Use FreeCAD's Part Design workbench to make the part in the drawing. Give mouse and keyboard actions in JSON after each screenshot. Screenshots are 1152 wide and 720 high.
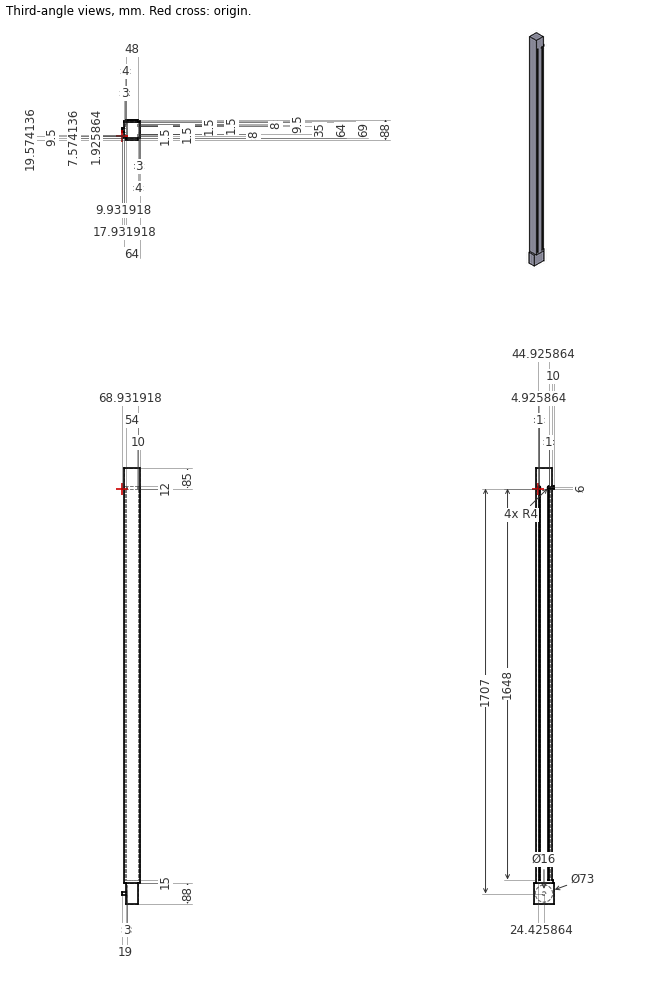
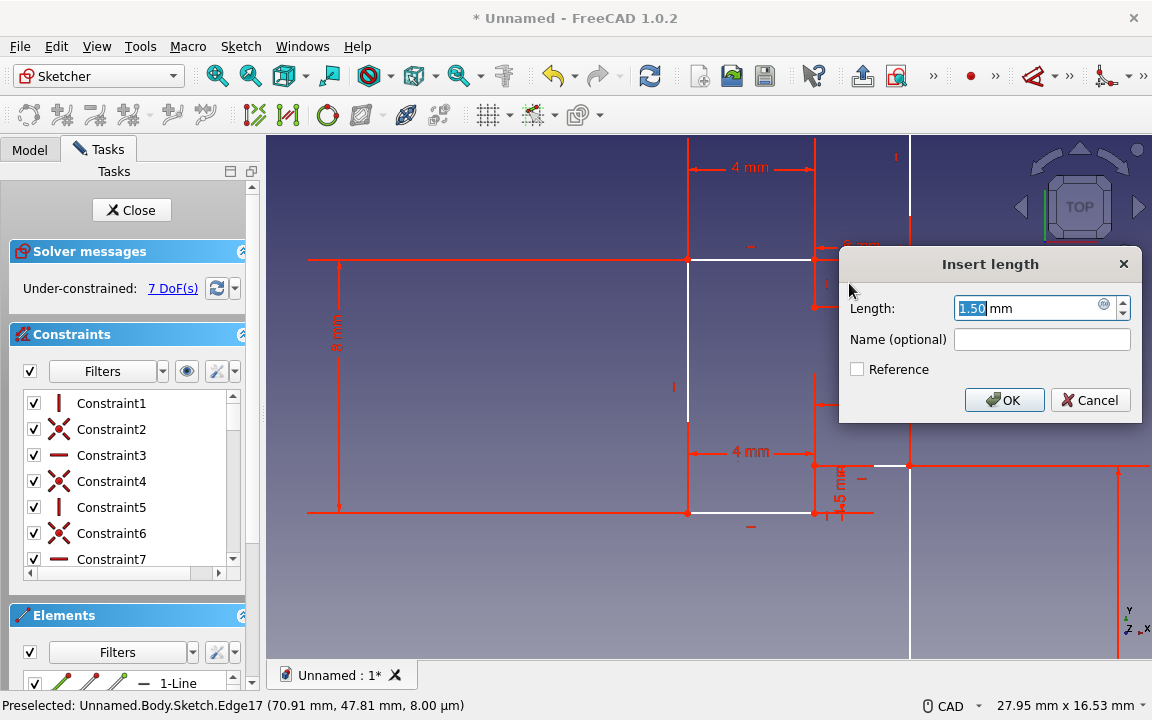
{"action": "type", "text": "1.5"}
{"action": "key", "text": "Return"}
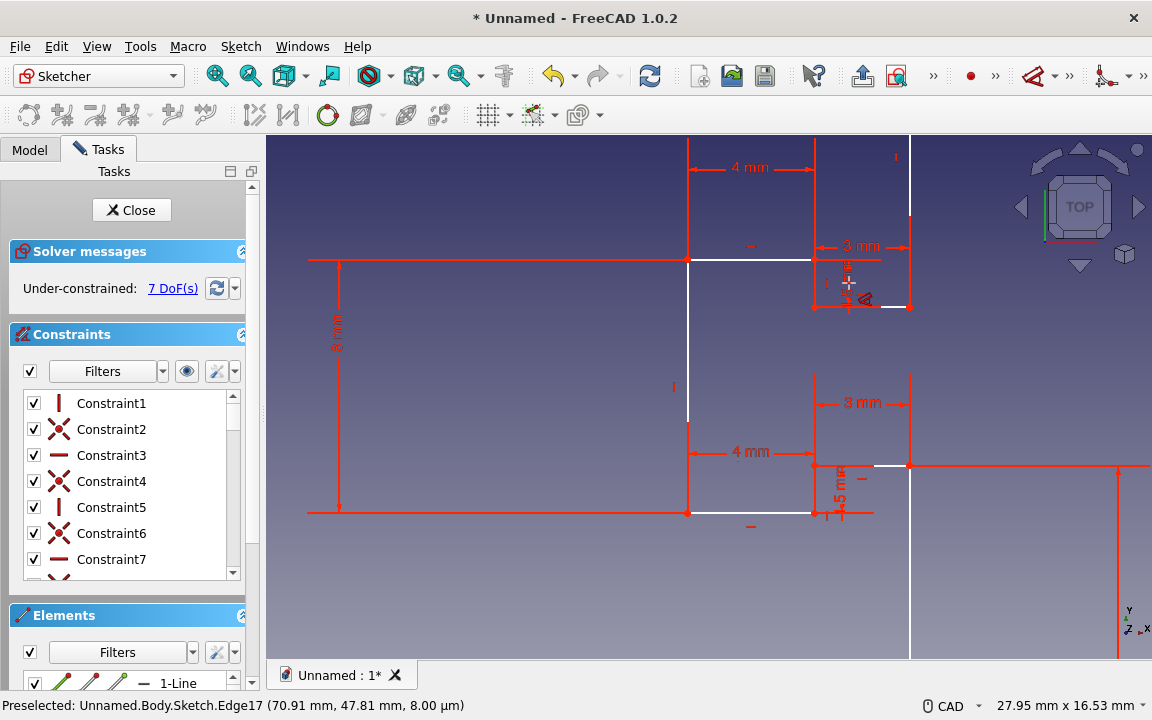
{"action": "scroll", "coordinate": [819, 274], "scroll_direction": "down", "scroll_amount": 9}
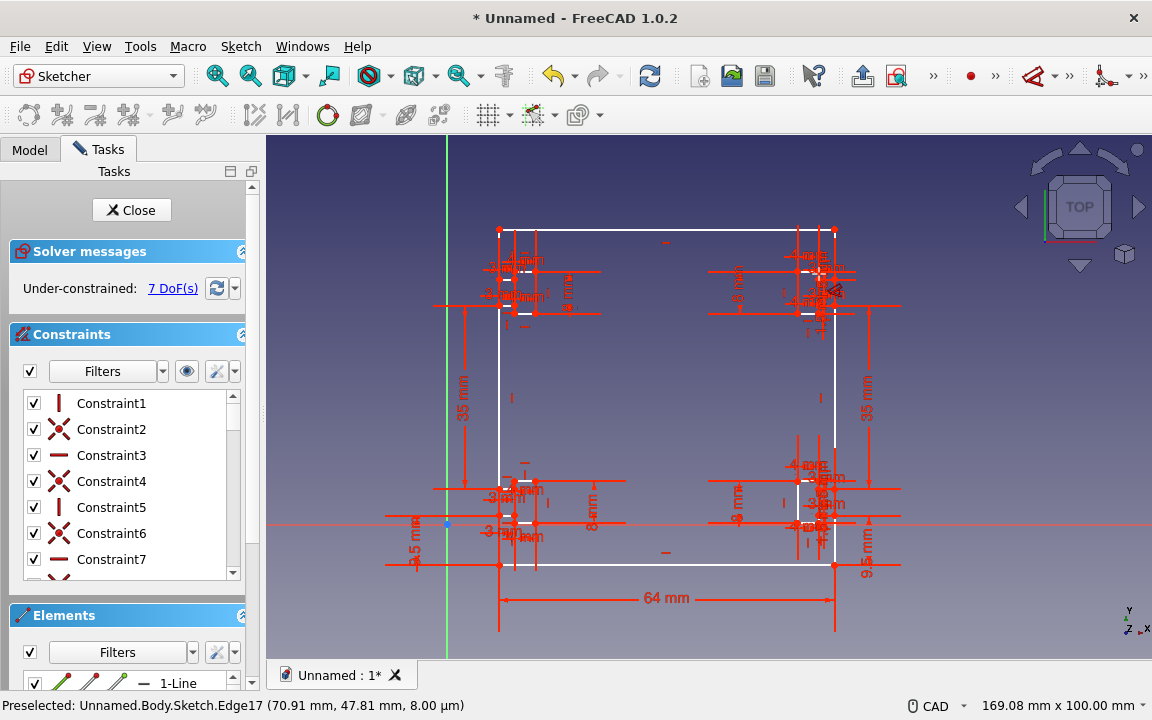
{"action": "left_click", "coordinate": [835, 265]}
{"action": "left_click", "coordinate": [893, 243]}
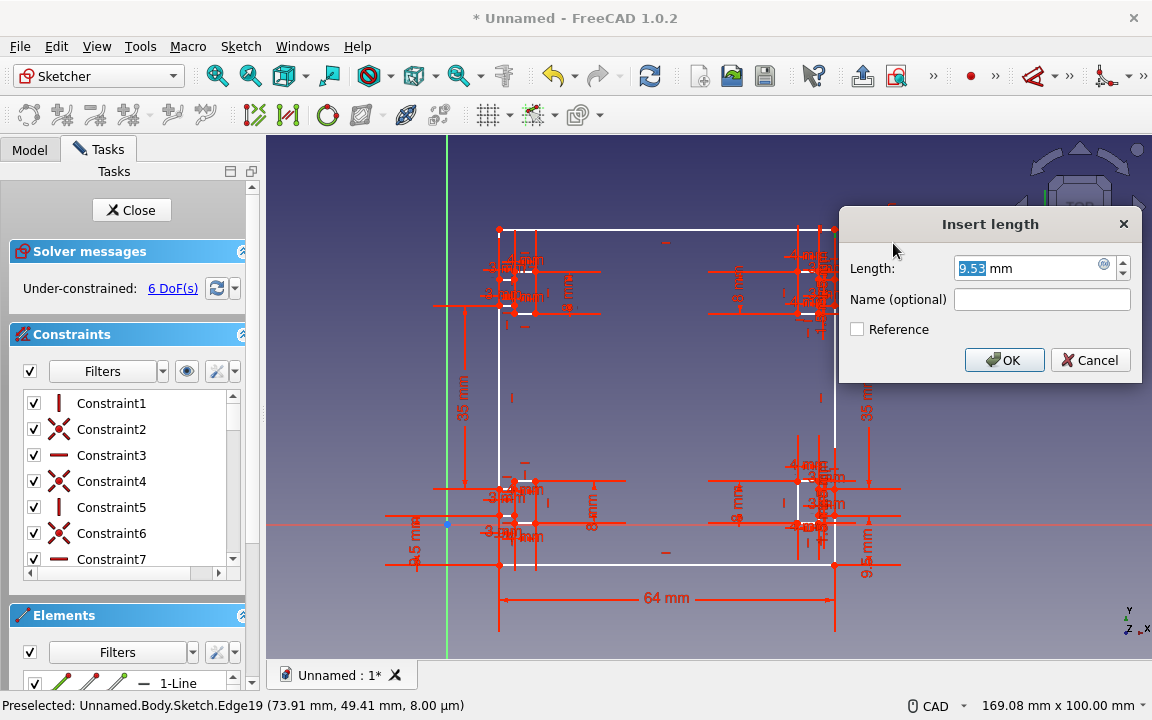
{"action": "type", "text": "9.5"}
{"action": "key", "text": "Return"}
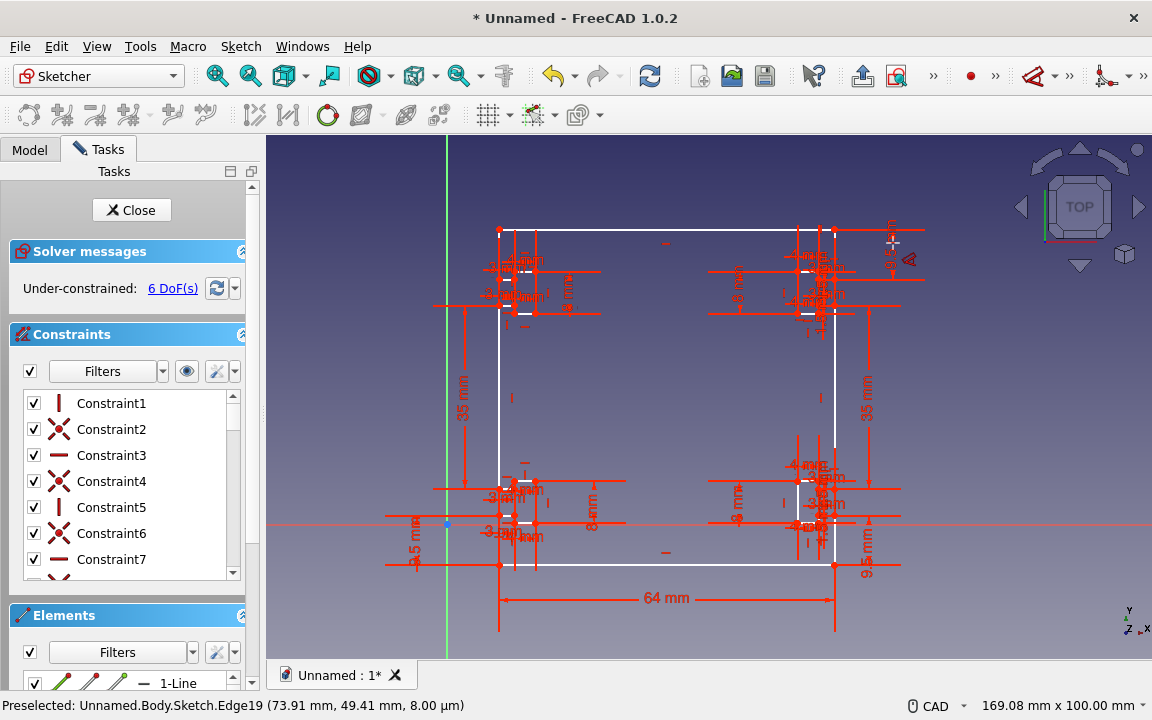
{"action": "left_click", "coordinate": [499, 245]}
{"action": "left_click", "coordinate": [465, 237]}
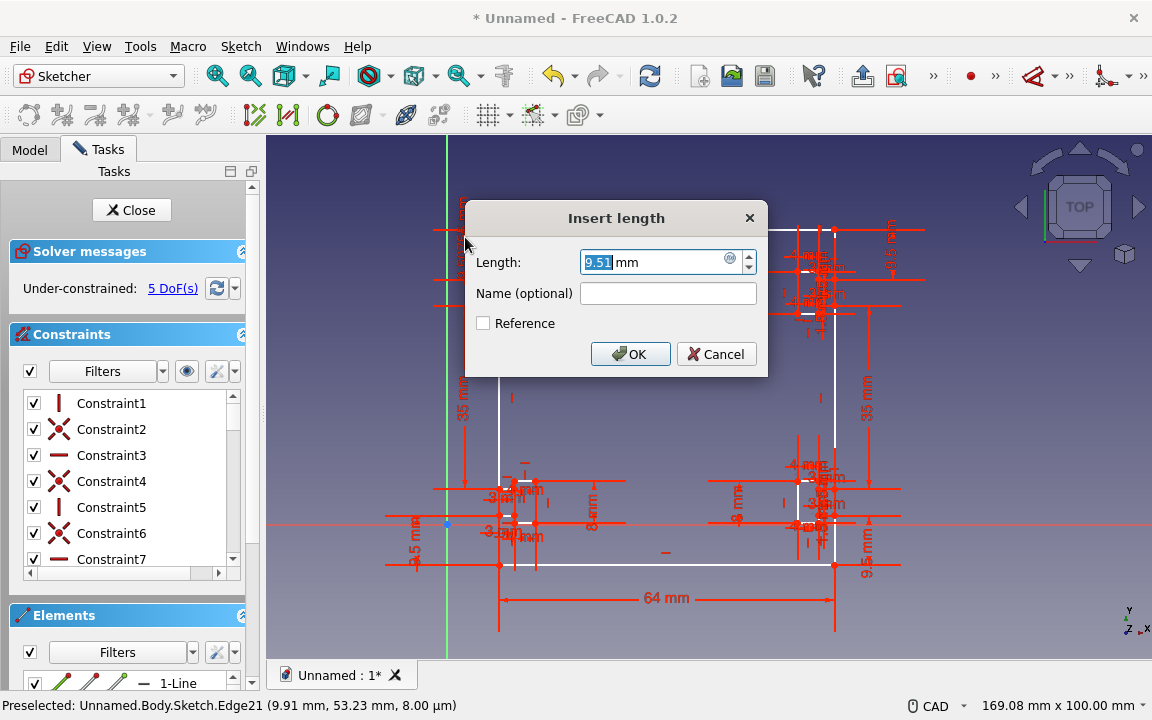
{"action": "type", "text": "9.5"}
{"action": "key", "text": "Return"}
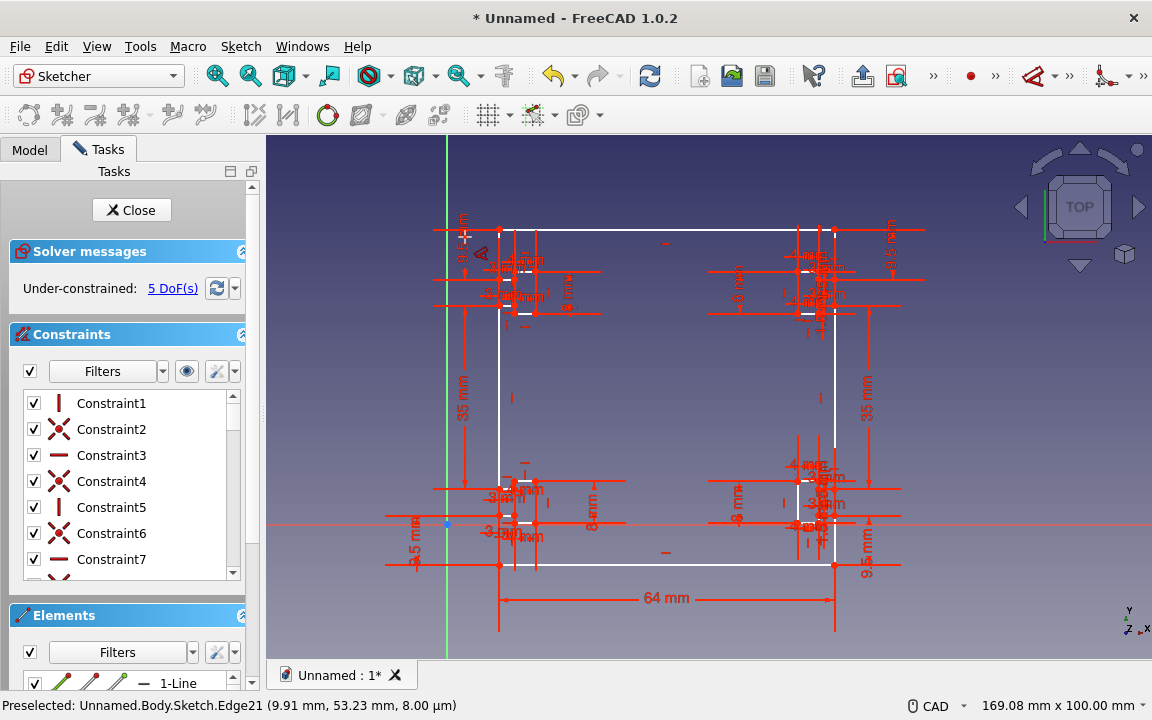
{"action": "scroll", "coordinate": [515, 276], "scroll_direction": "up", "scroll_amount": 9}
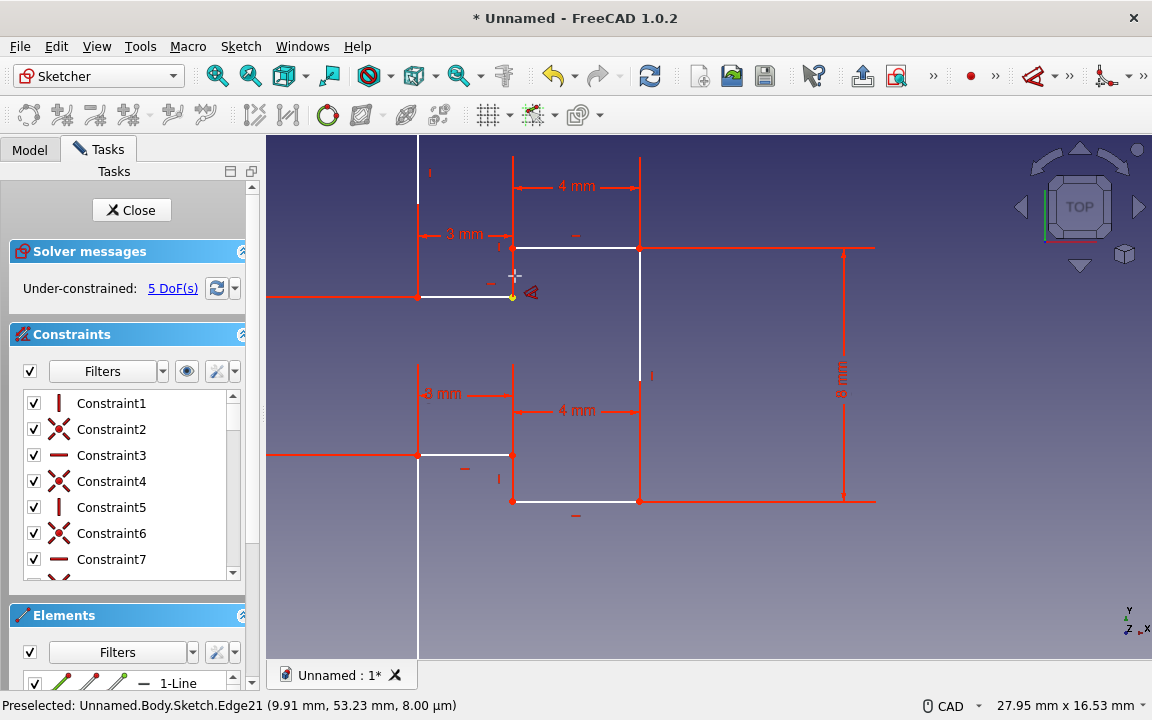
{"action": "left_click", "coordinate": [513, 273]}
{"action": "left_click", "coordinate": [479, 273]}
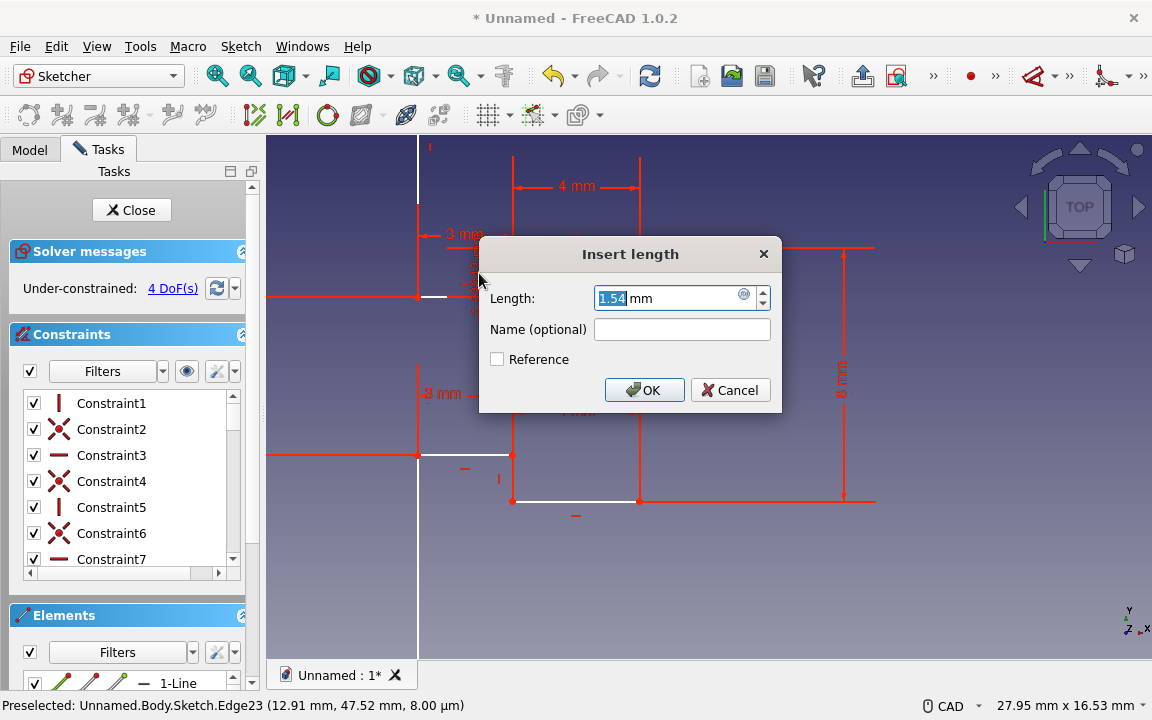
{"action": "type", "text": "1.5"}
{"action": "key", "text": "Return"}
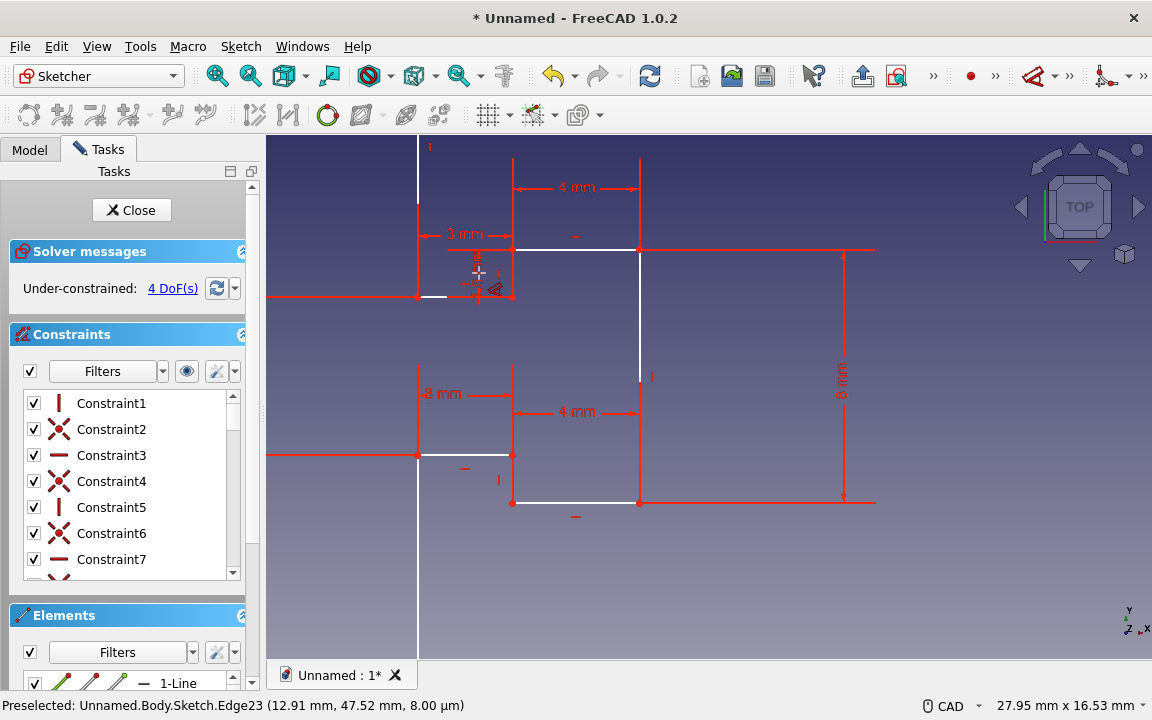
{"action": "left_click", "coordinate": [513, 489]}
{"action": "left_click", "coordinate": [479, 479]}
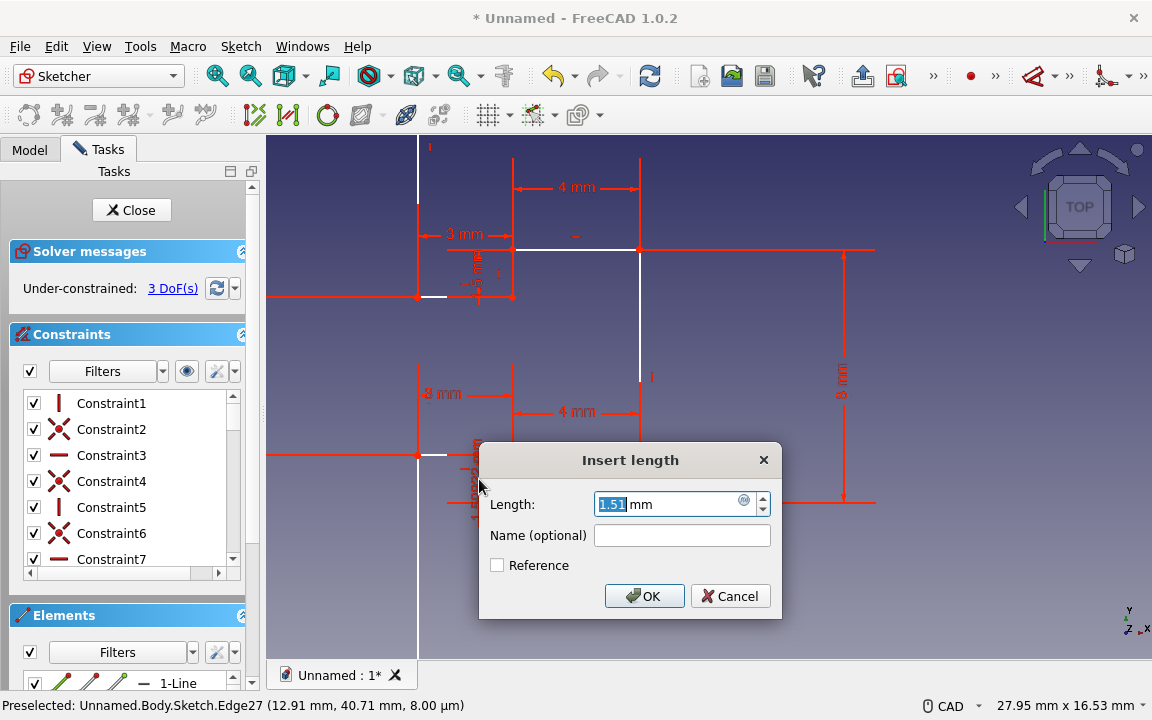
{"action": "type", "text": "1.5"}
{"action": "key", "text": "Return"}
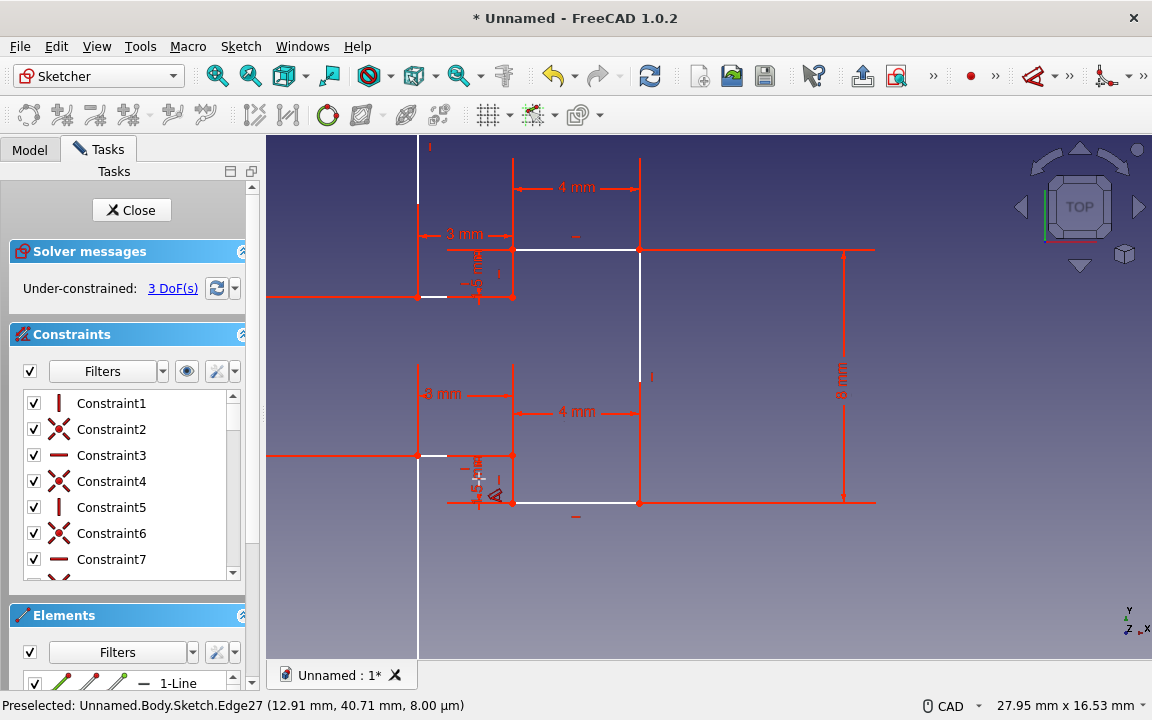
{"action": "scroll", "coordinate": [515, 276], "scroll_direction": "down", "scroll_amount": 9}